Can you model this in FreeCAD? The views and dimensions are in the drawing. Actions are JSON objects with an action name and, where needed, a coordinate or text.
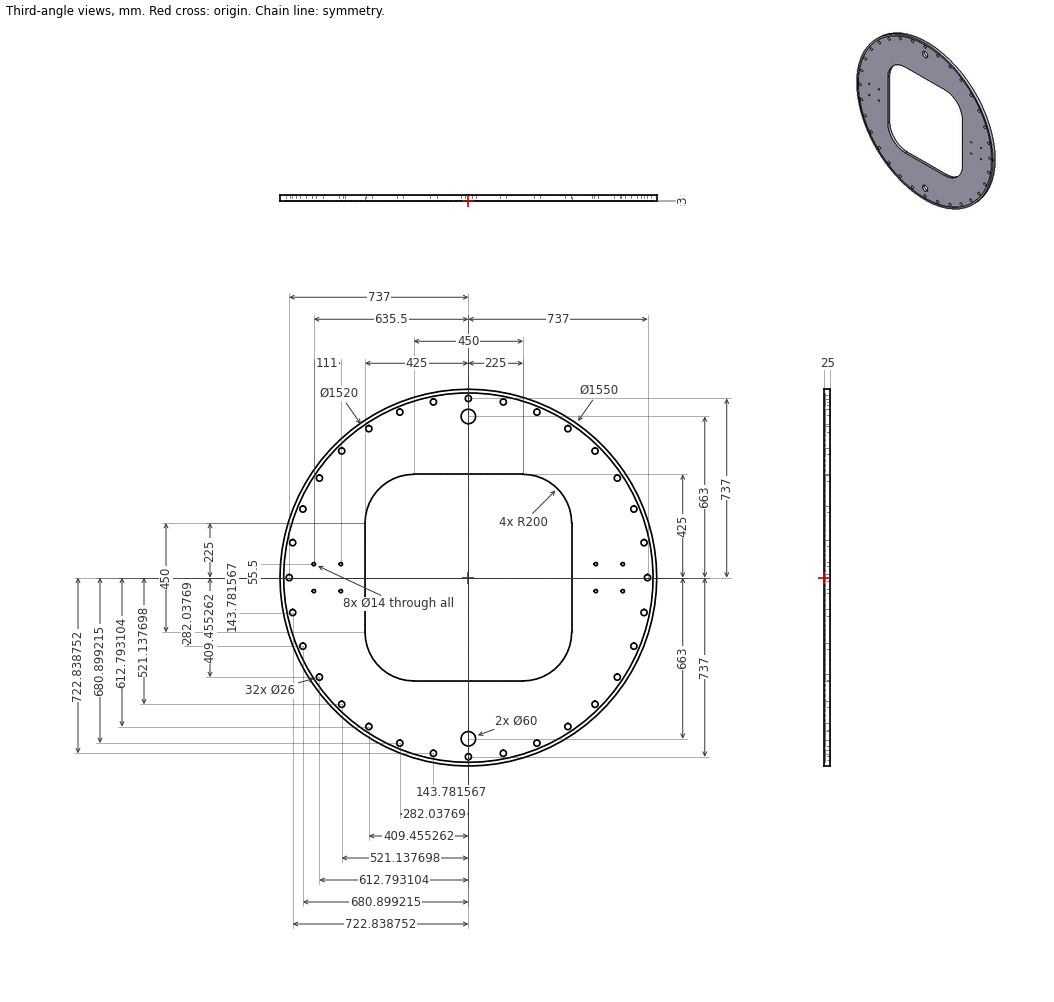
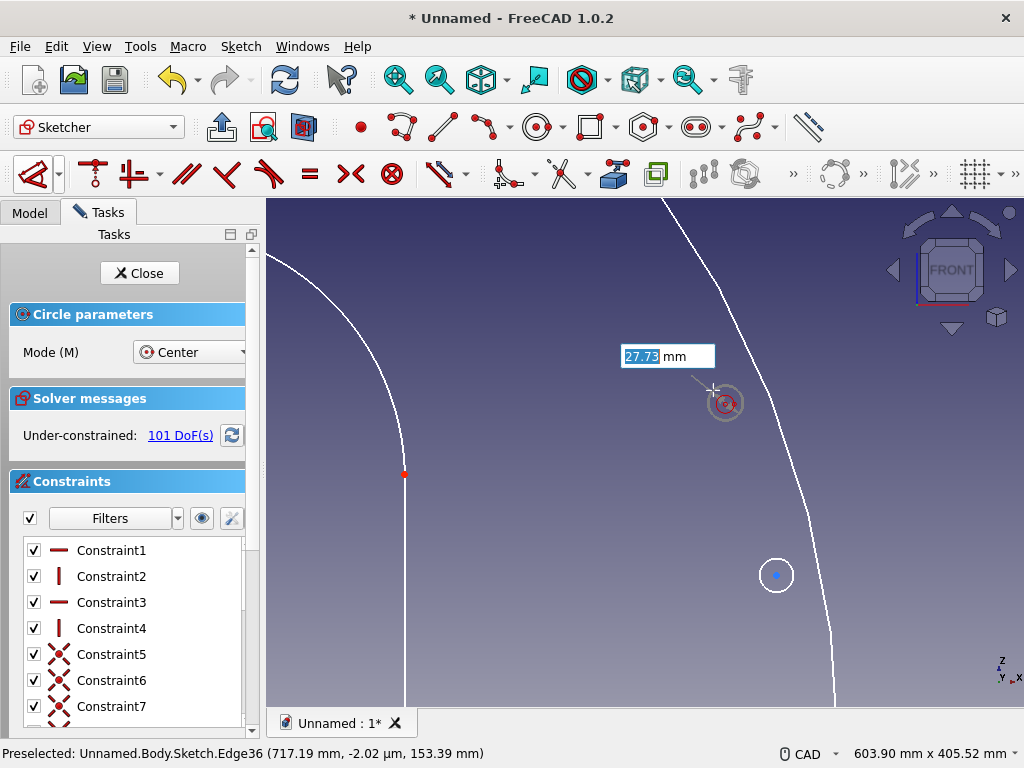
{"action": "left_click", "coordinate": [713, 388]}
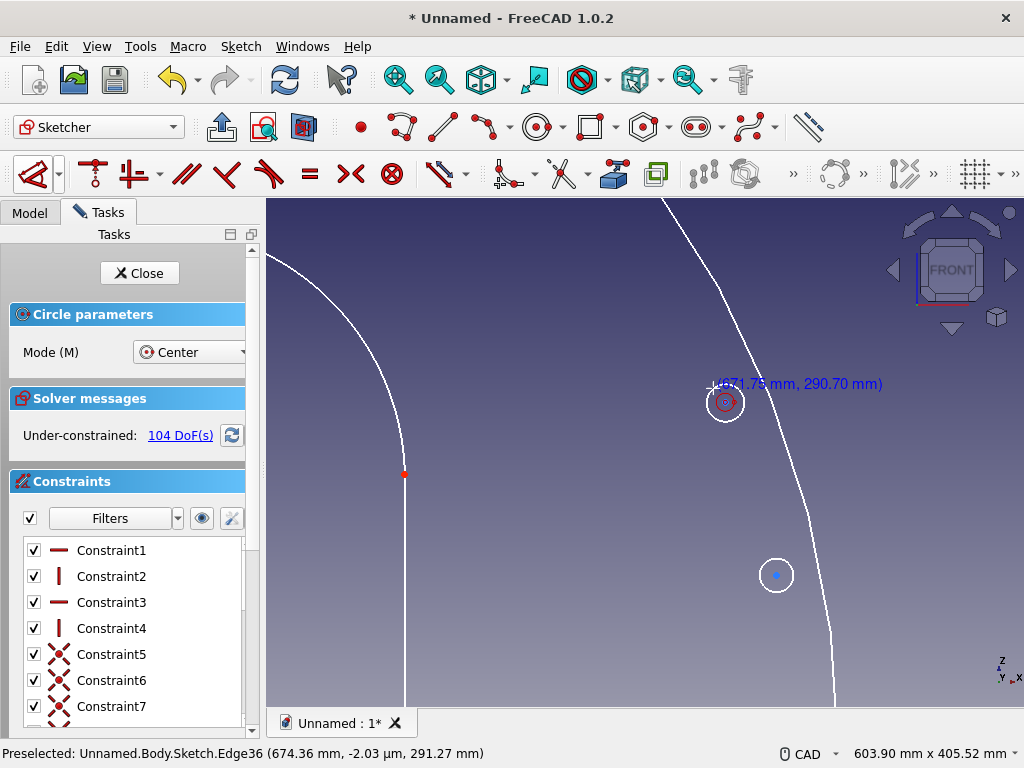
{"action": "scroll", "coordinate": [716, 393], "scroll_direction": "down", "scroll_amount": 9}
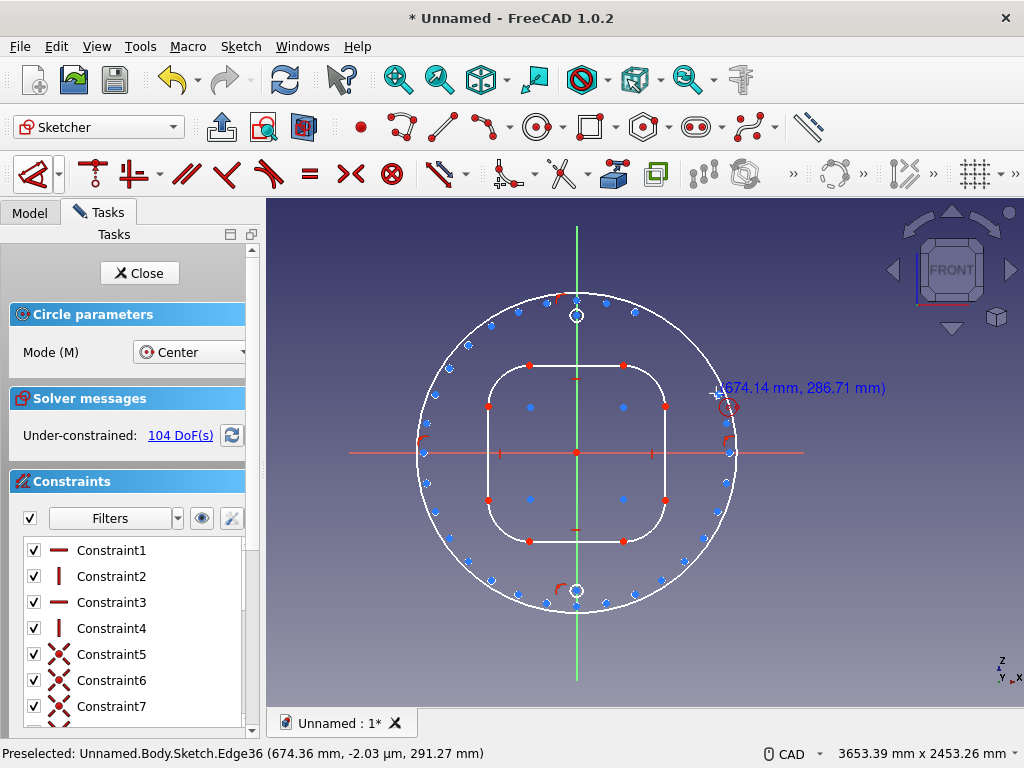
{"action": "scroll", "coordinate": [685, 345], "scroll_direction": "up", "scroll_amount": 11}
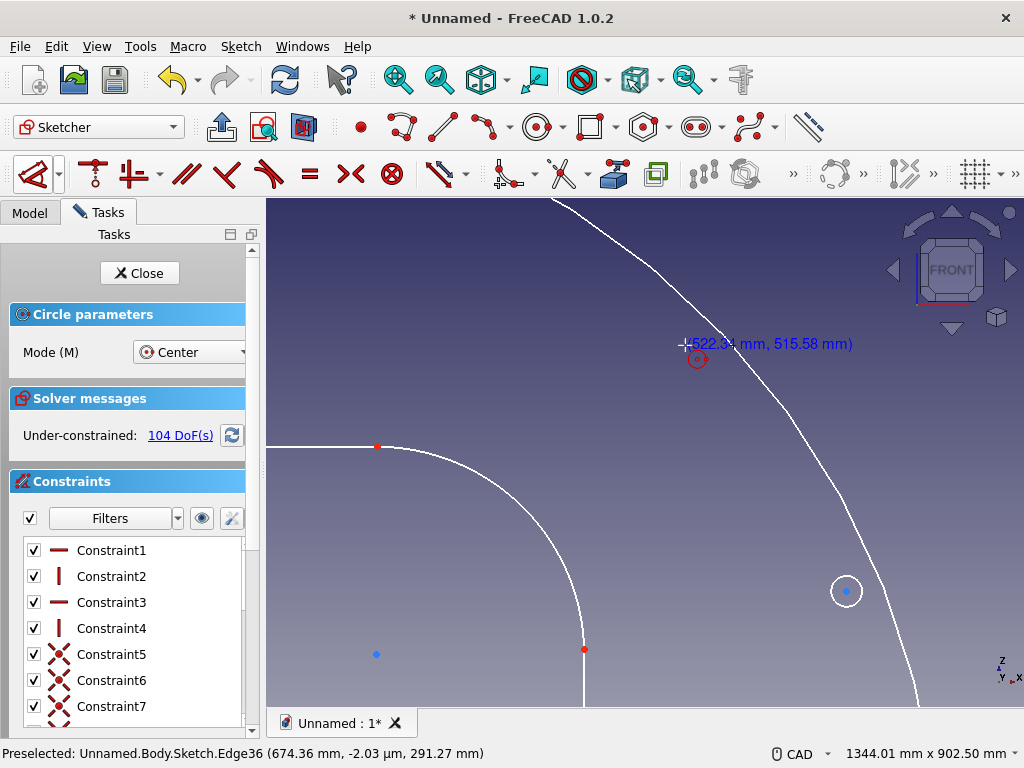
{"action": "scroll", "coordinate": [685, 345], "scroll_direction": "down", "scroll_amount": 11}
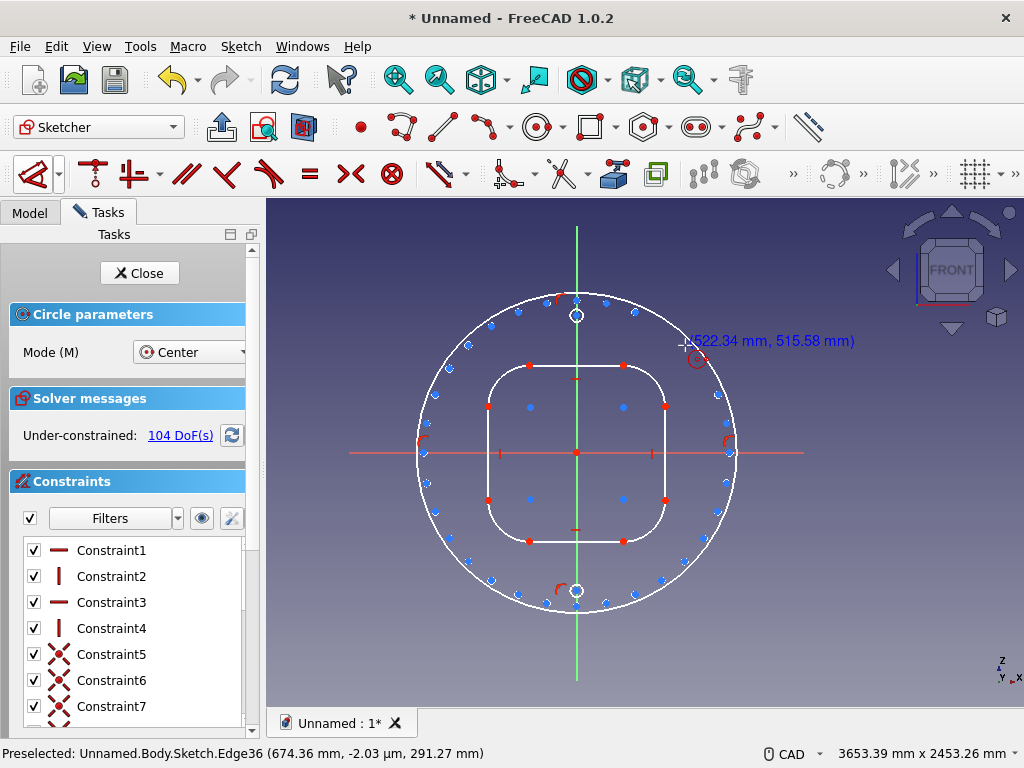
{"action": "scroll", "coordinate": [685, 345], "scroll_direction": "up", "scroll_amount": 4}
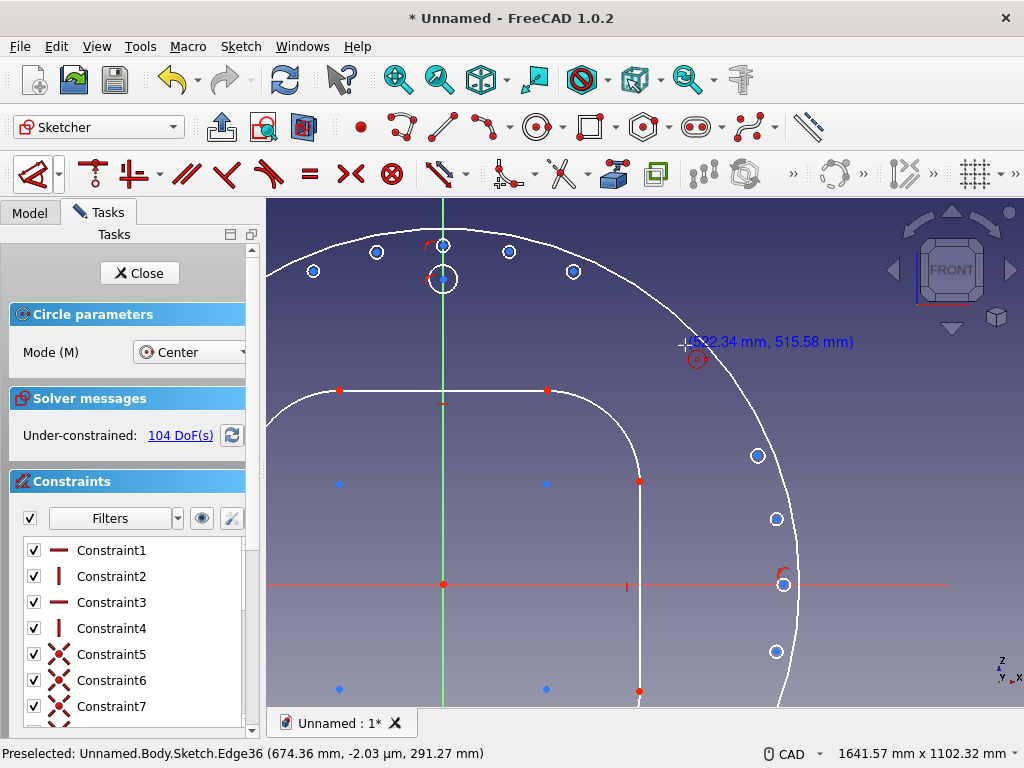
{"action": "left_click", "coordinate": [684, 344]}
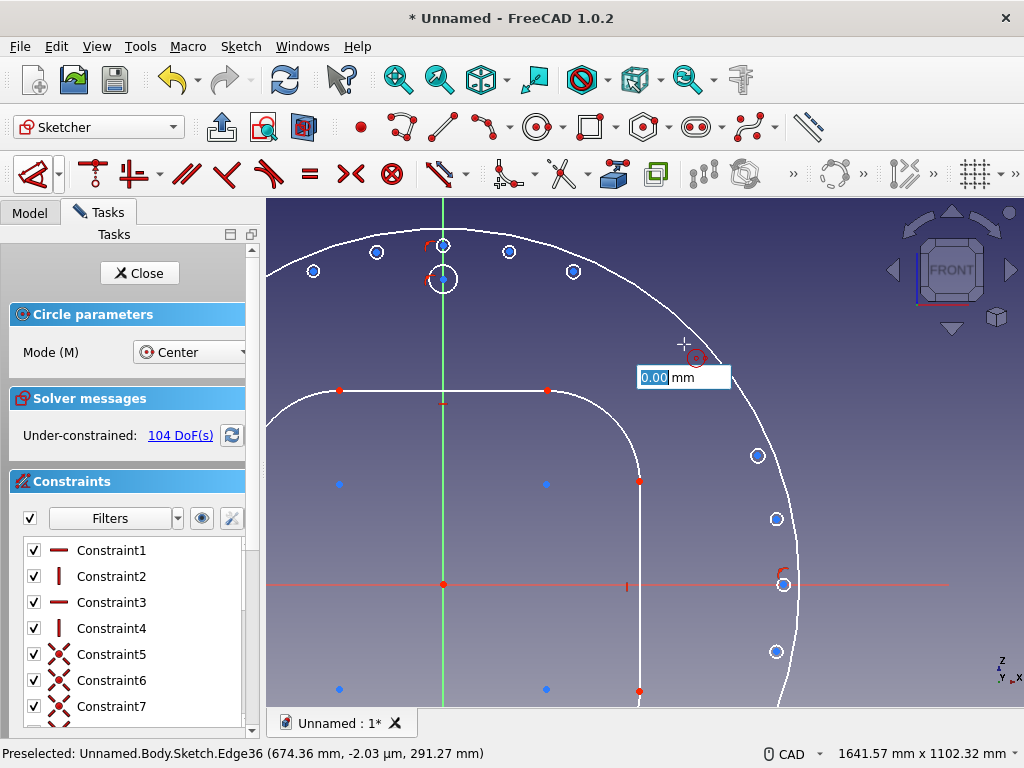
{"action": "scroll", "coordinate": [680, 340], "scroll_direction": "up", "scroll_amount": 5}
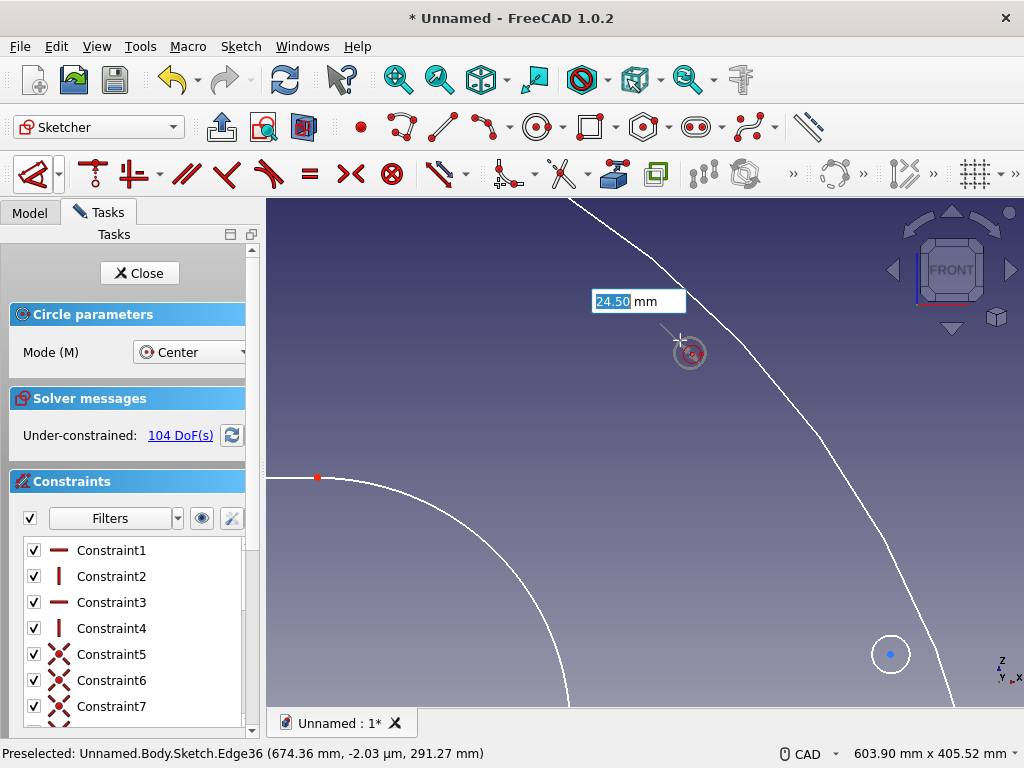
{"action": "left_click", "coordinate": [678, 340]}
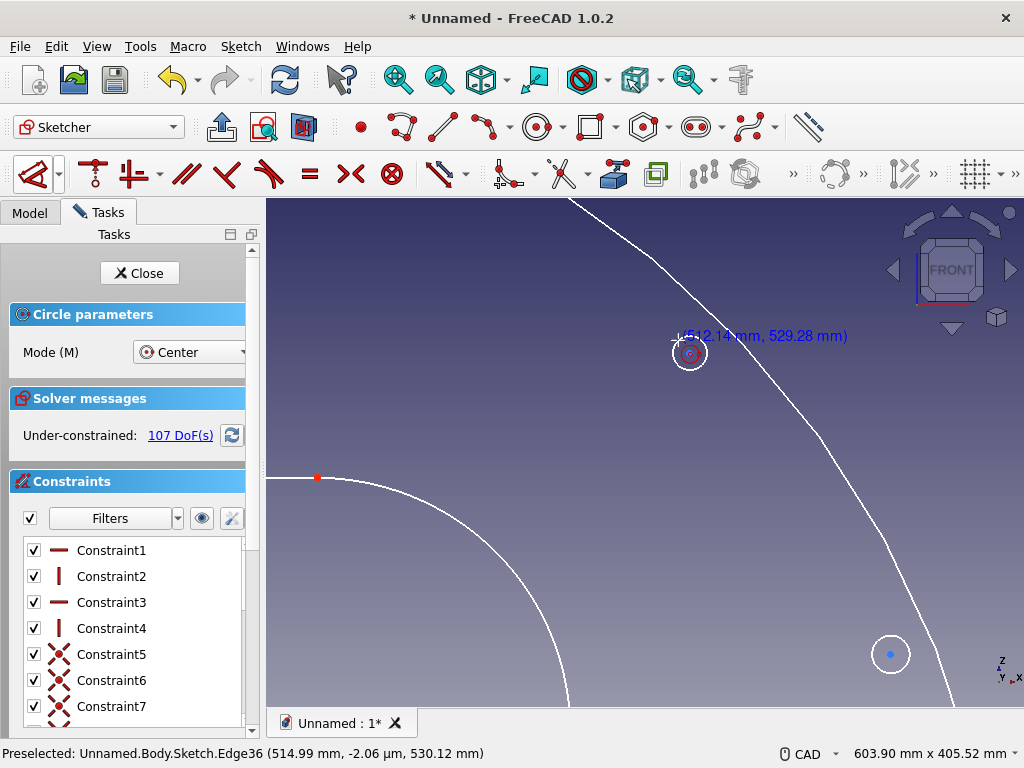
{"action": "scroll", "coordinate": [549, 236], "scroll_direction": "up", "scroll_amount": 2}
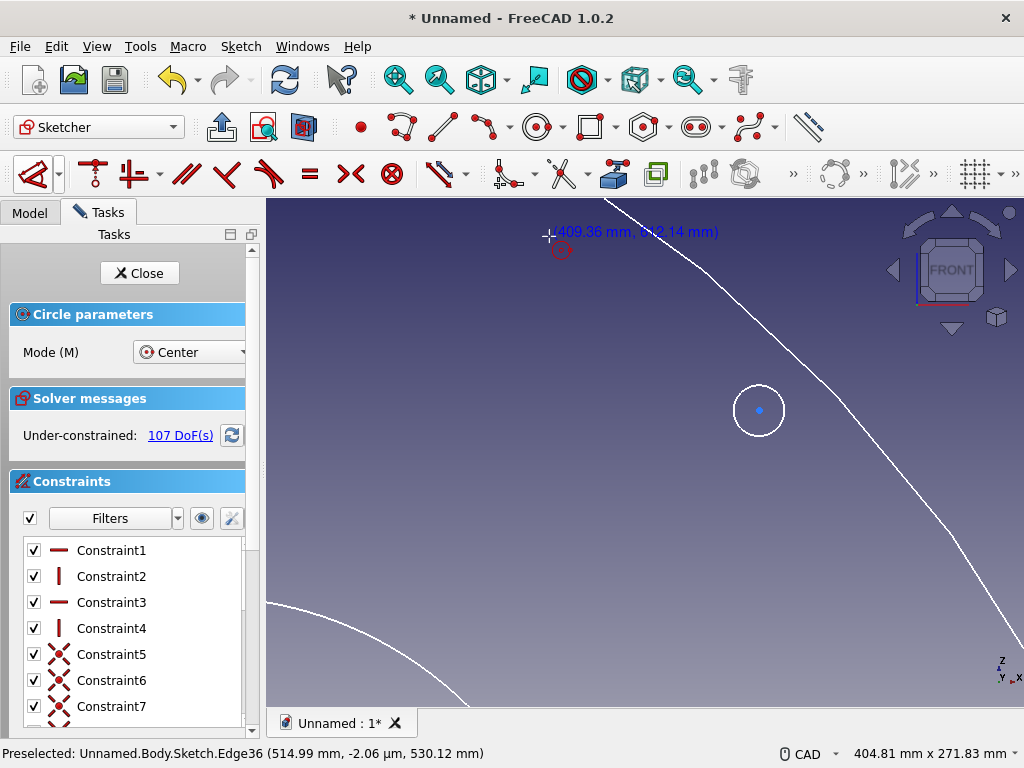
{"action": "scroll", "coordinate": [675, 336], "scroll_direction": "down", "scroll_amount": 11}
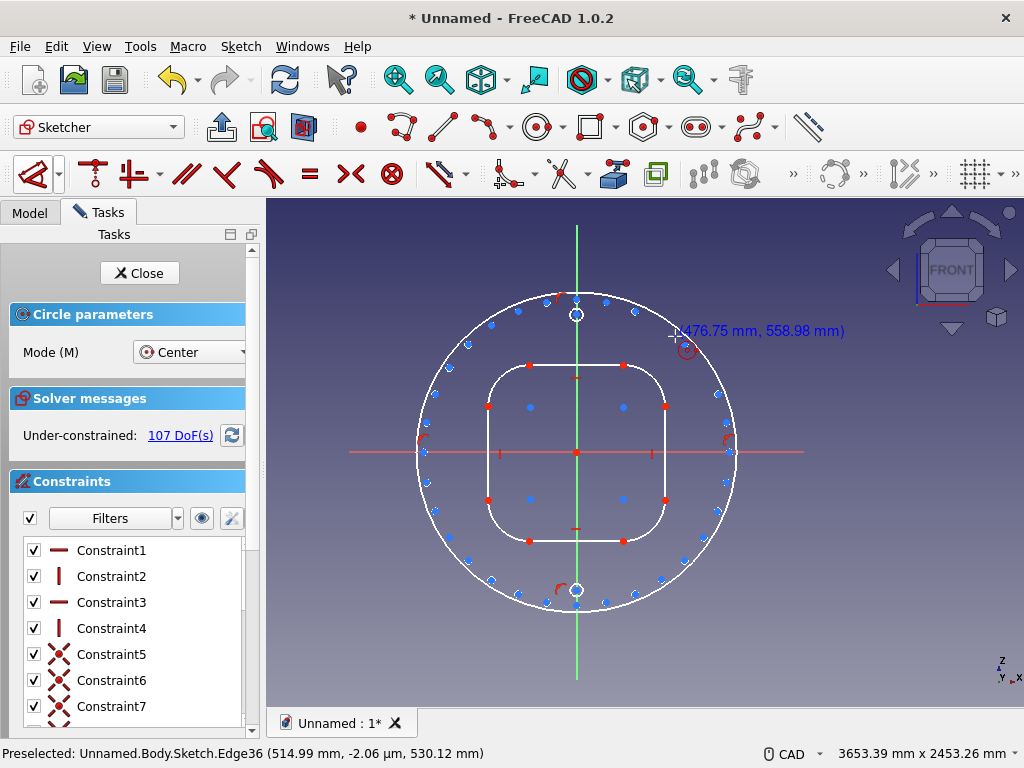
{"action": "scroll", "coordinate": [662, 325], "scroll_direction": "up", "scroll_amount": 4}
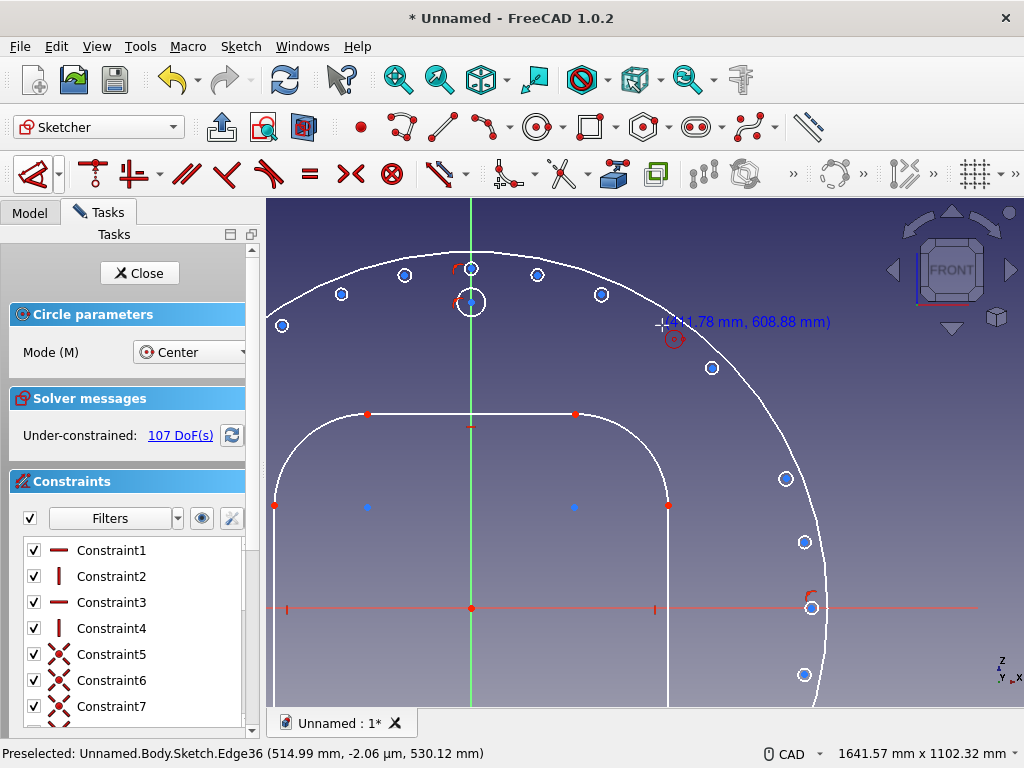
{"action": "left_click", "coordinate": [660, 325]}